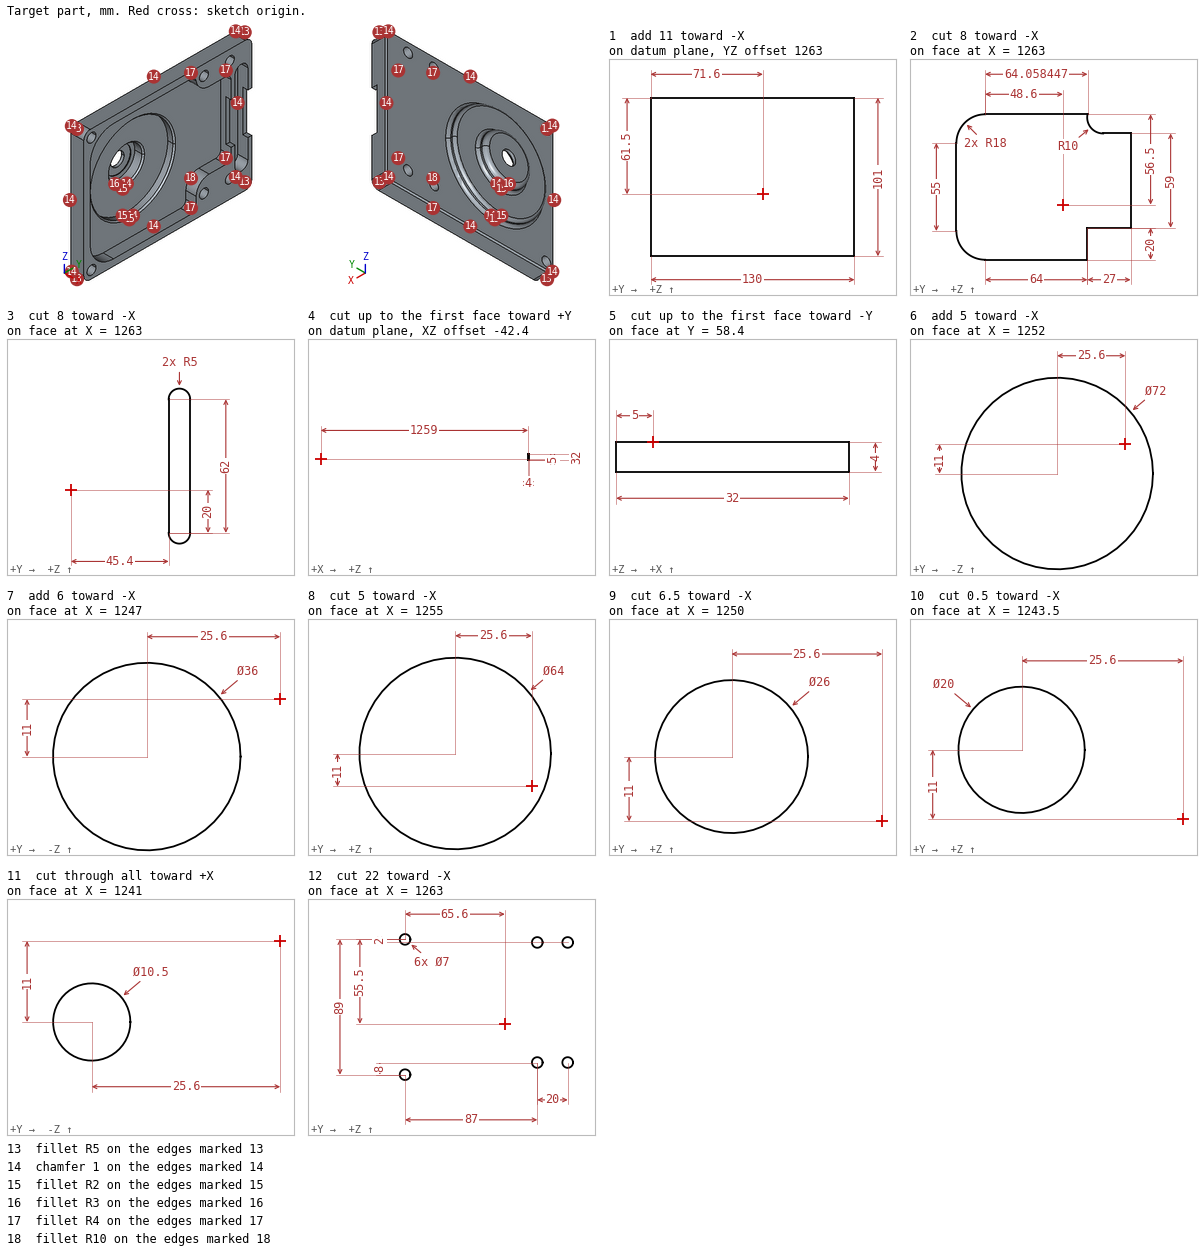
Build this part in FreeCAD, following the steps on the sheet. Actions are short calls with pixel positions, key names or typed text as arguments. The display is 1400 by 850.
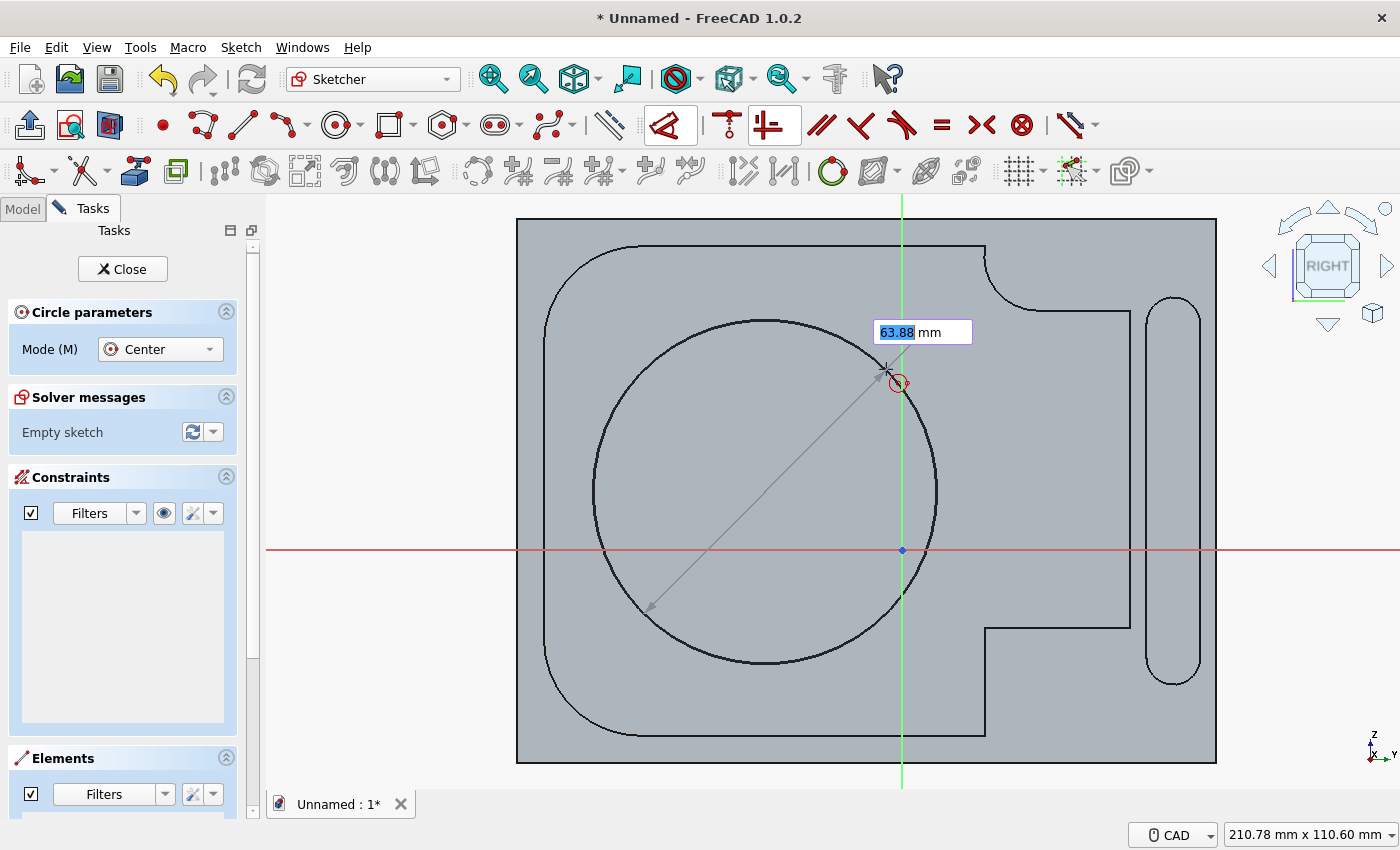
text(64)
key(Return)
key(Escape)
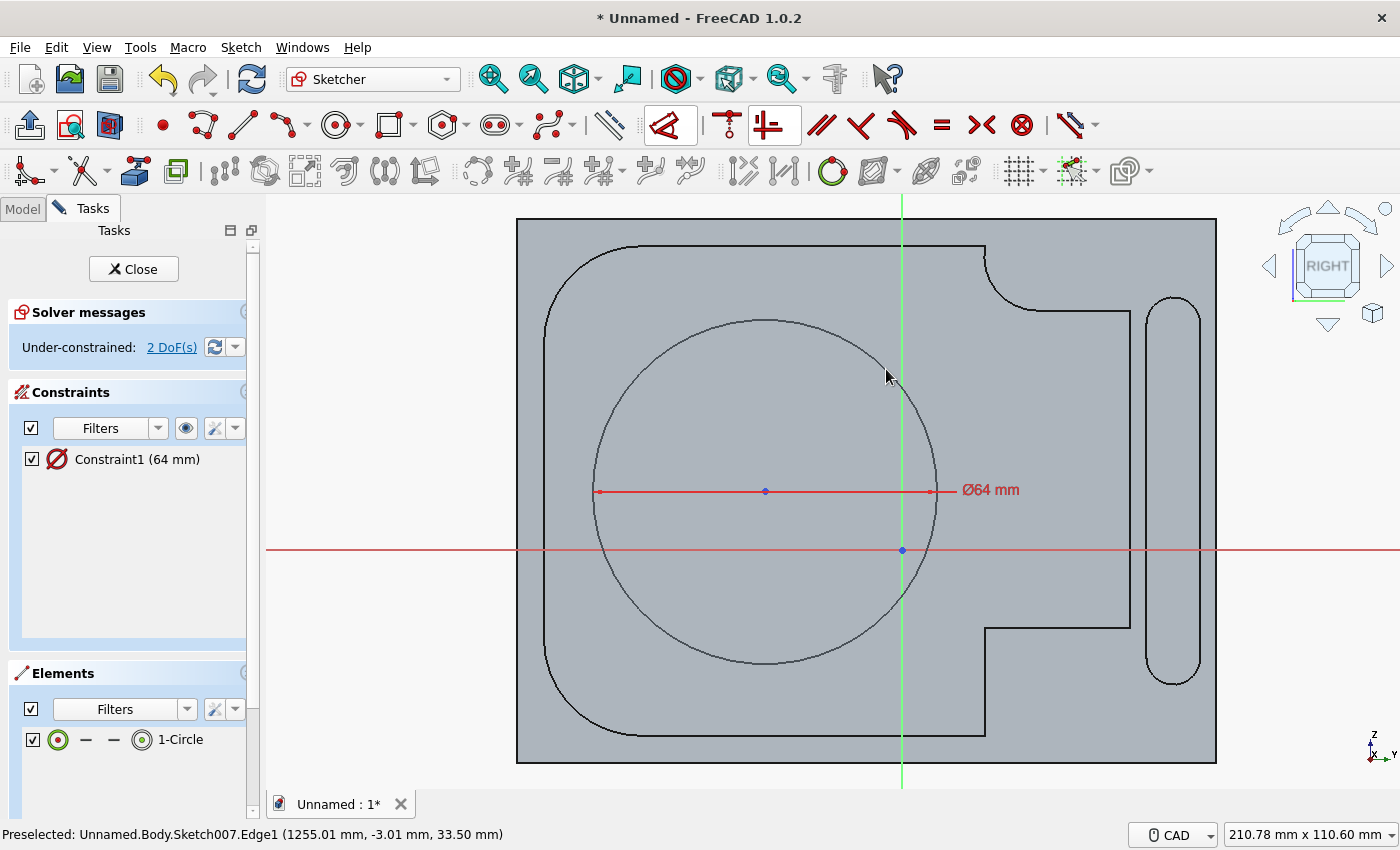
click(765, 492)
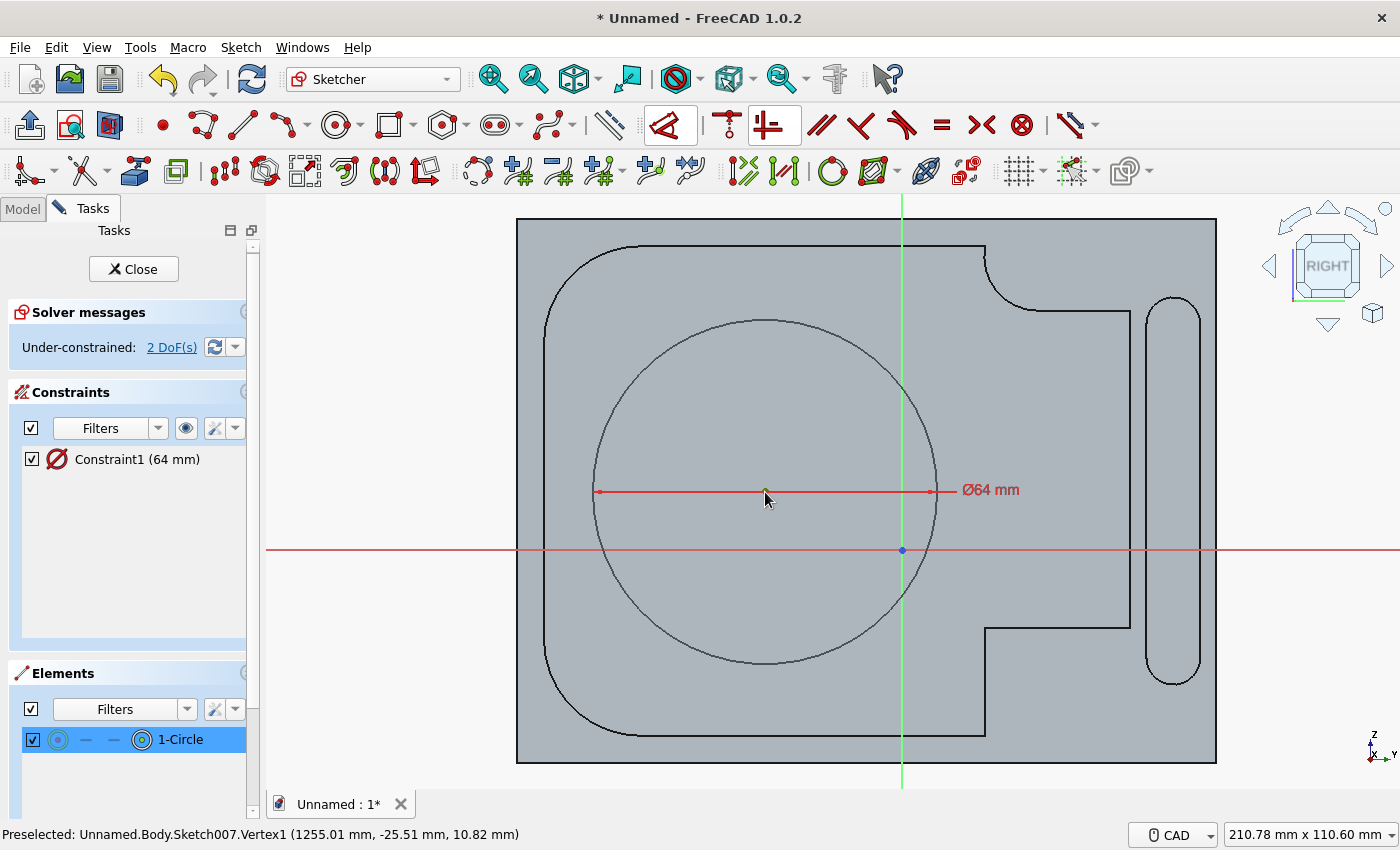
key(i)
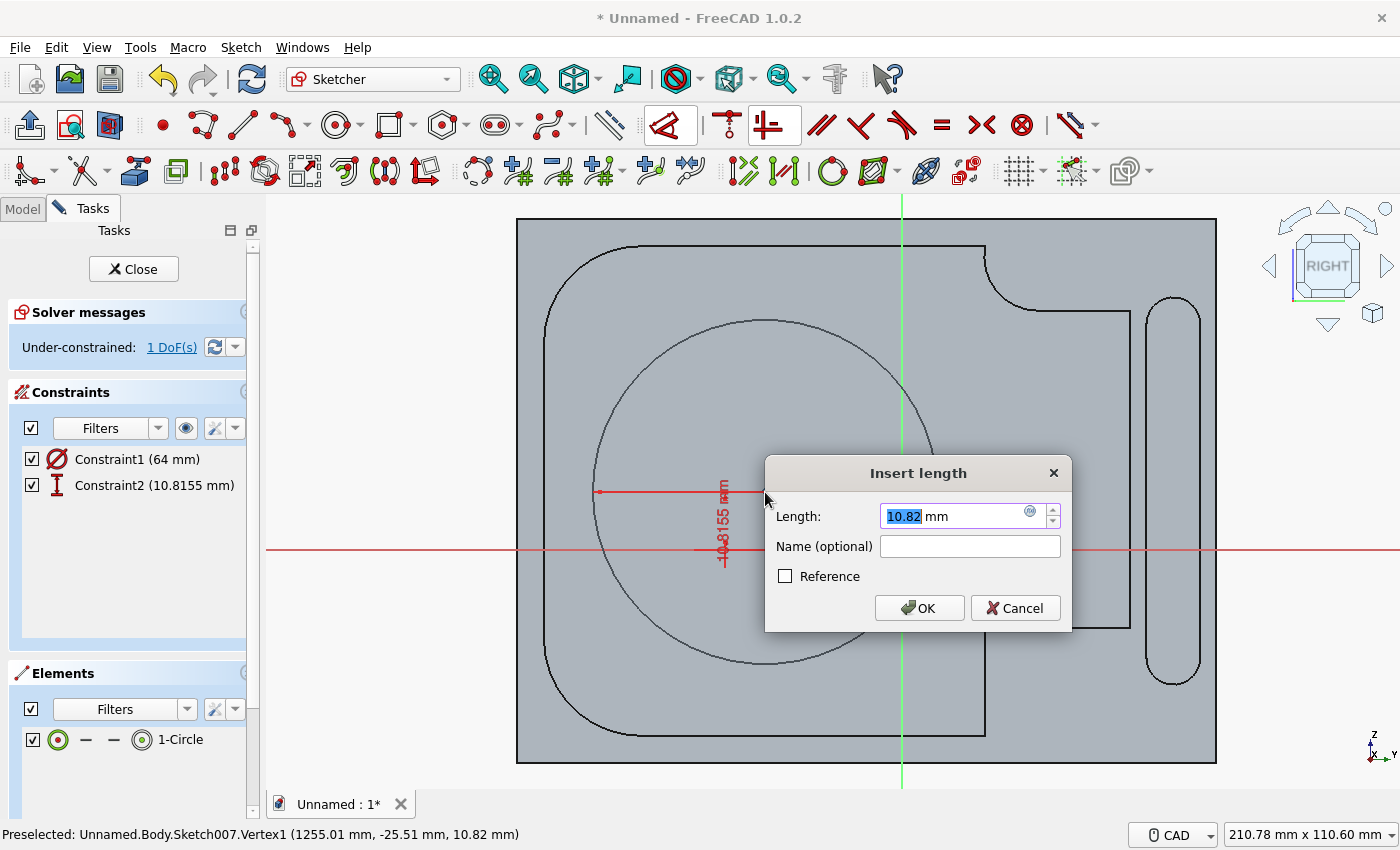
text(11)
key(Return)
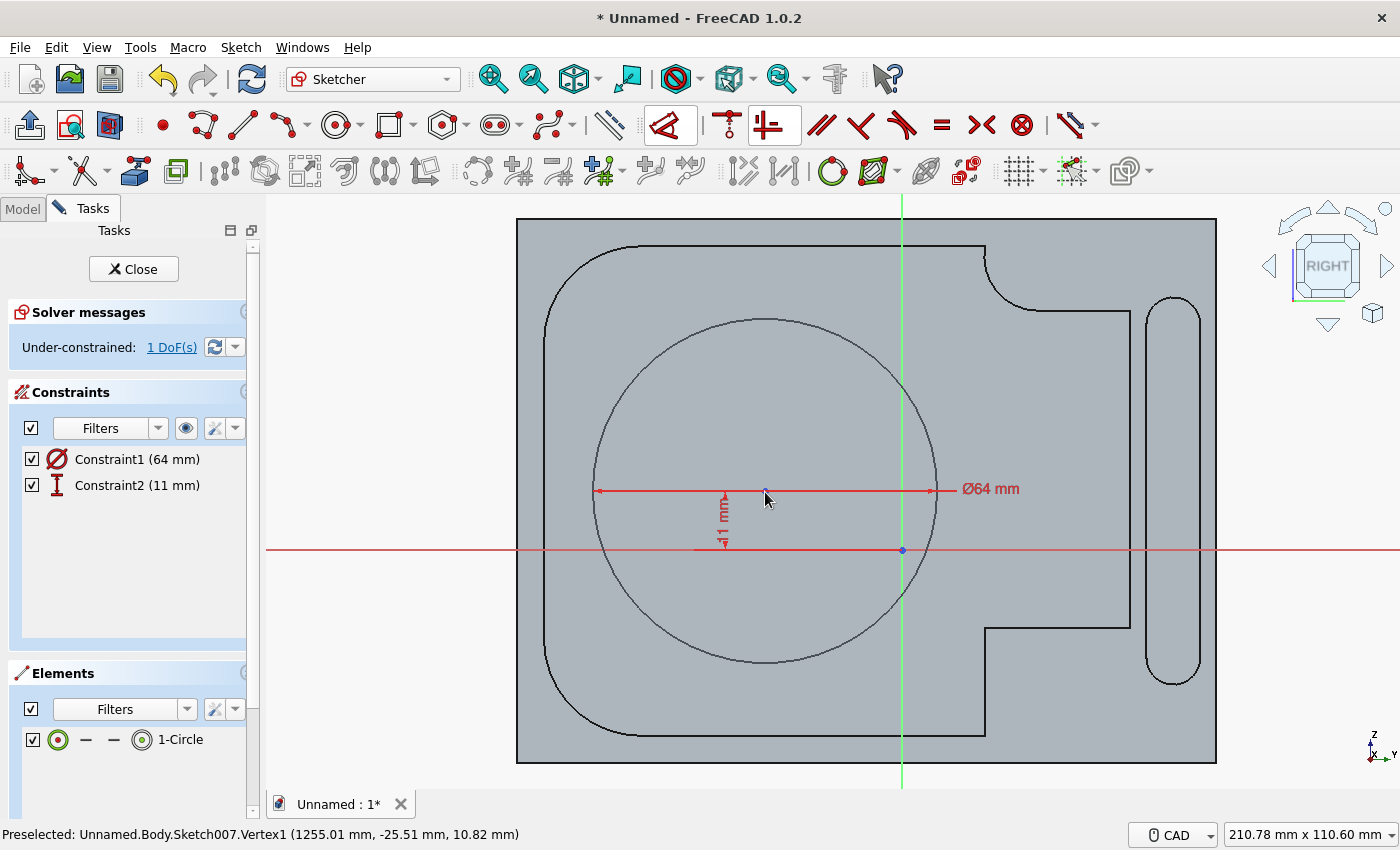
click(765, 491)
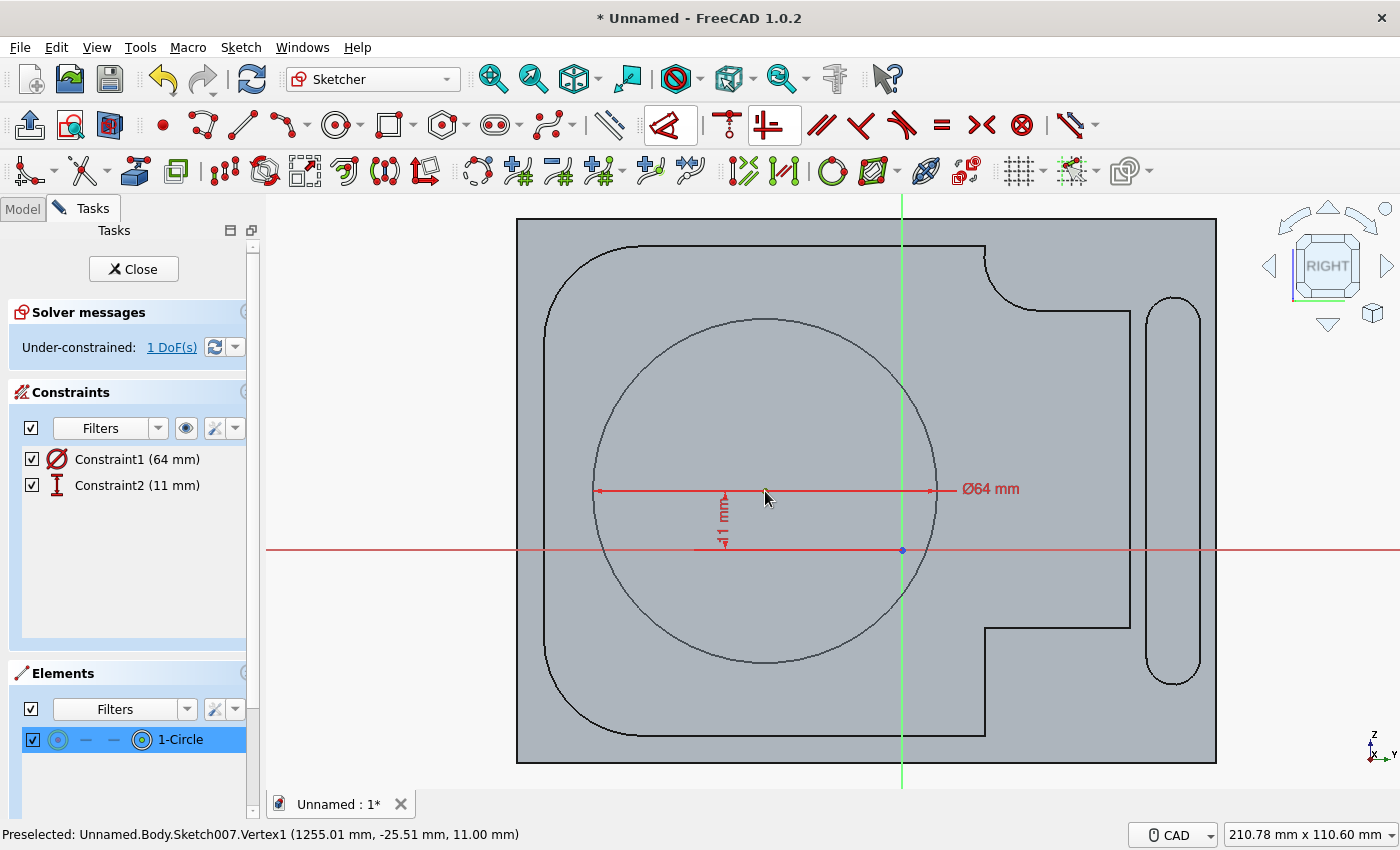
key(l)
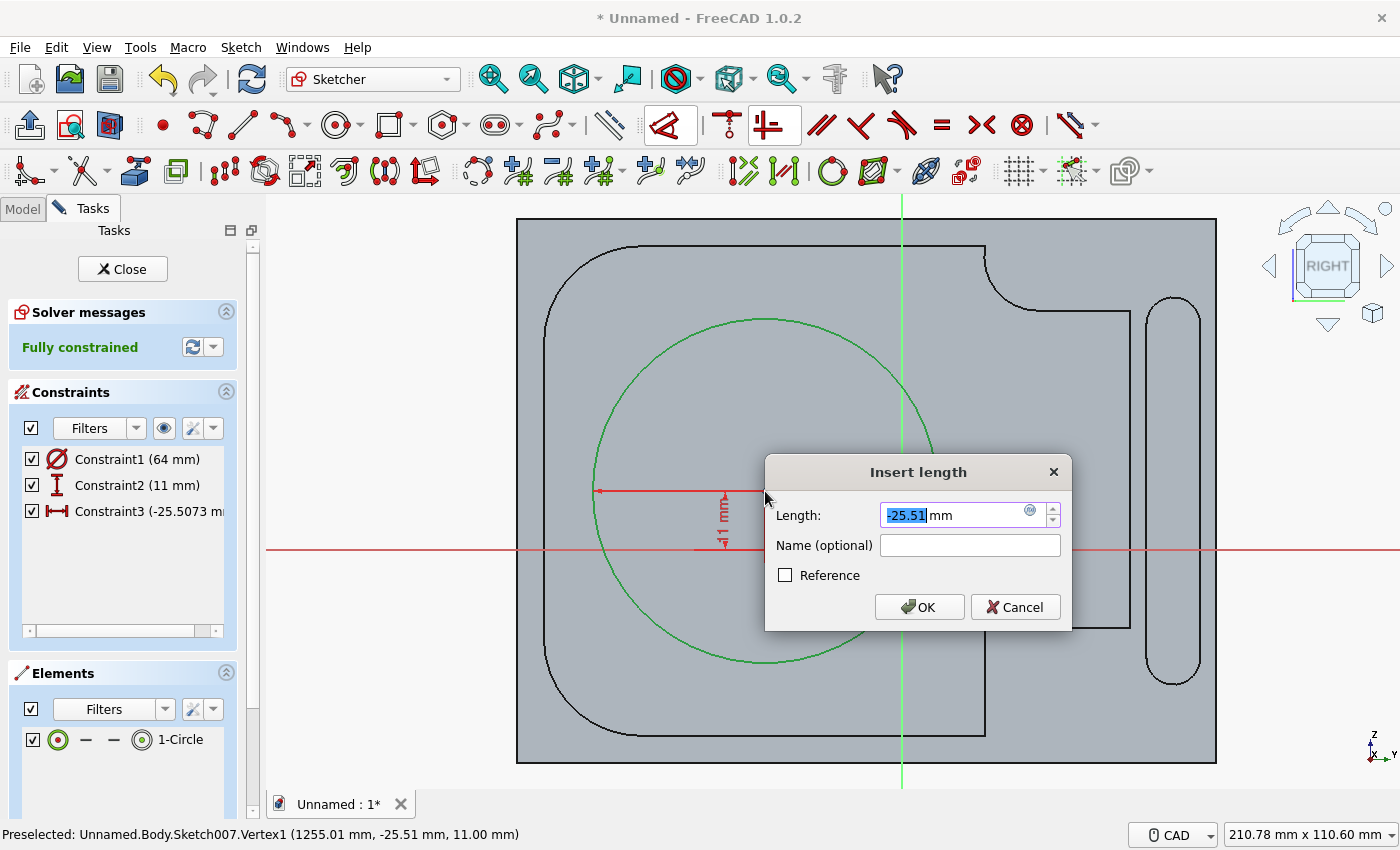
text(-25.6)
key(Return)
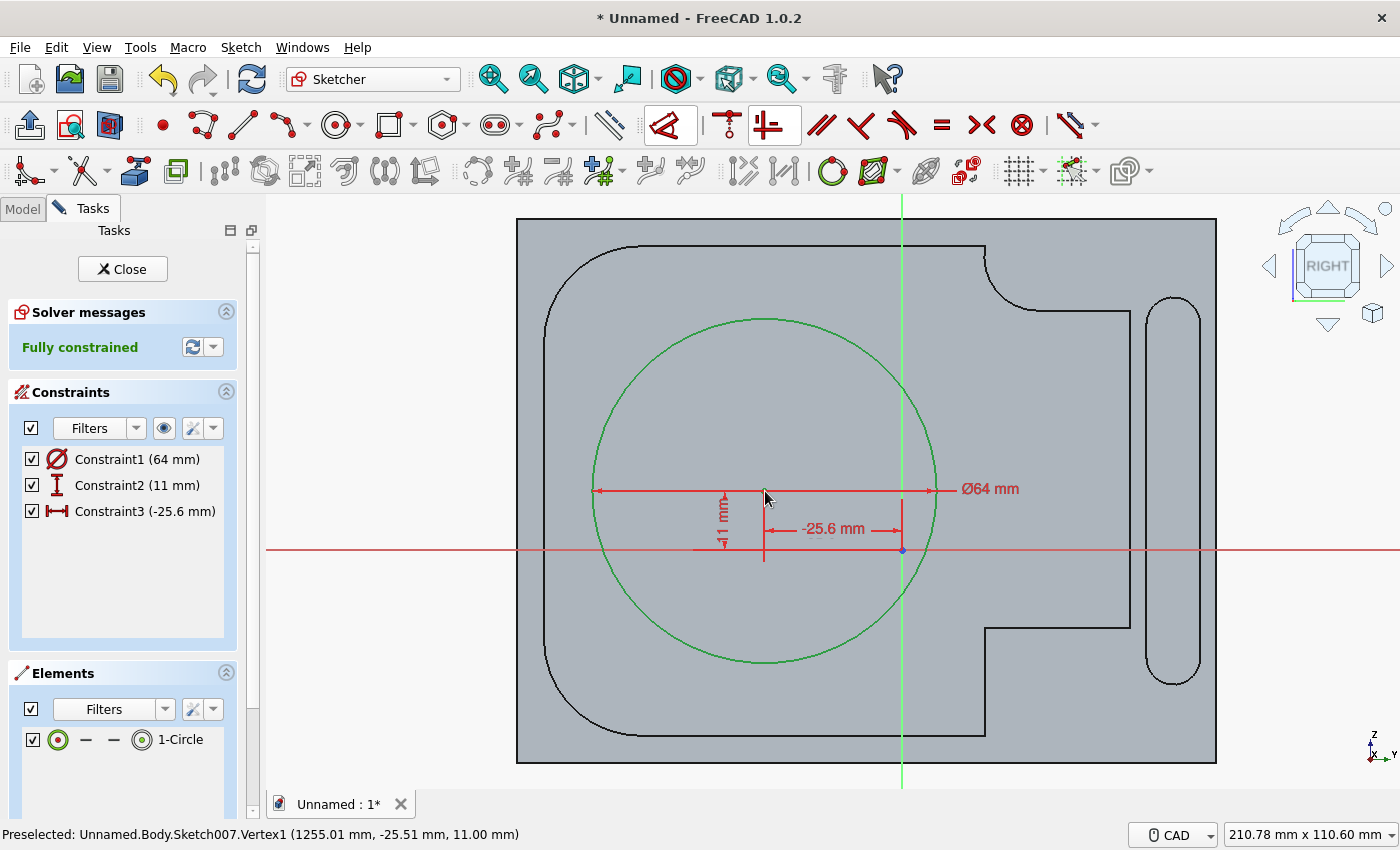
click(123, 269)